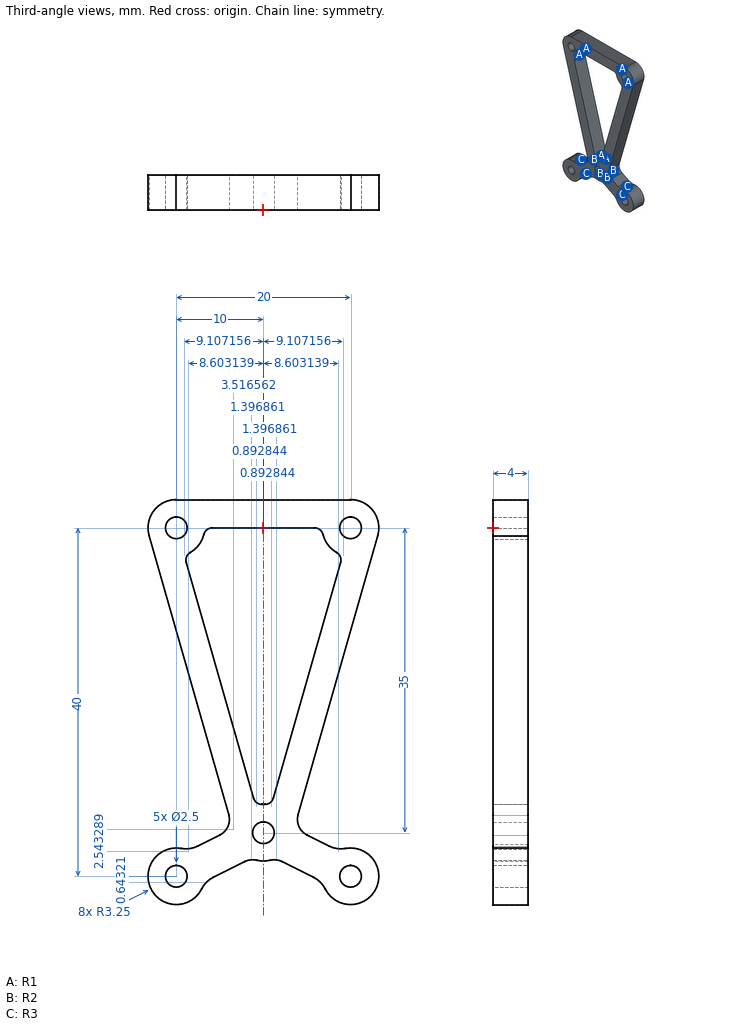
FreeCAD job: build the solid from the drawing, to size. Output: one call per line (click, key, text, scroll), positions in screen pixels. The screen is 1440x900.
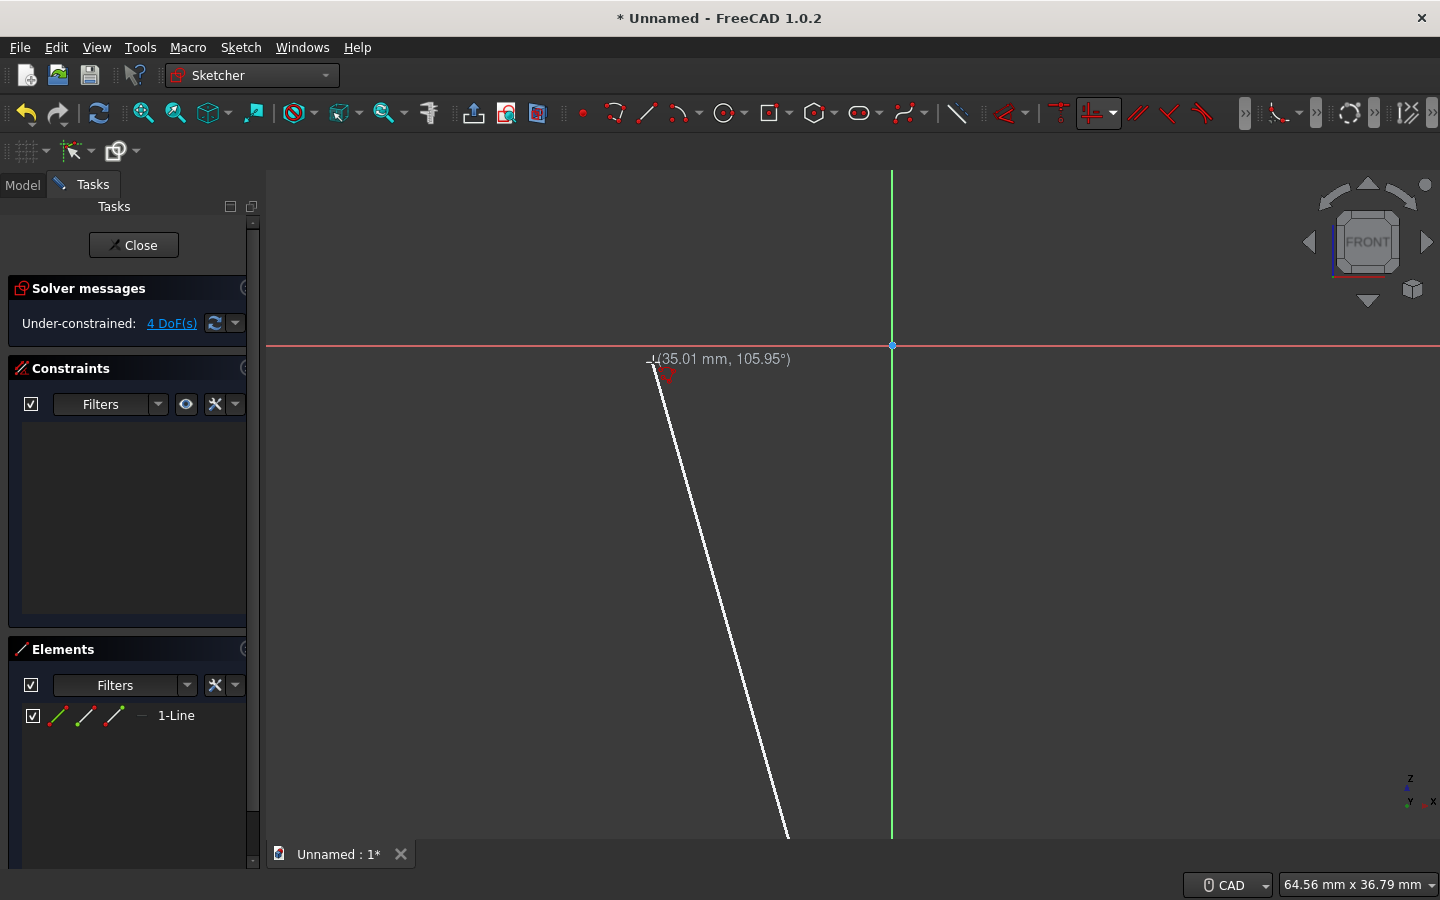
click(653, 362)
right_click(653, 362)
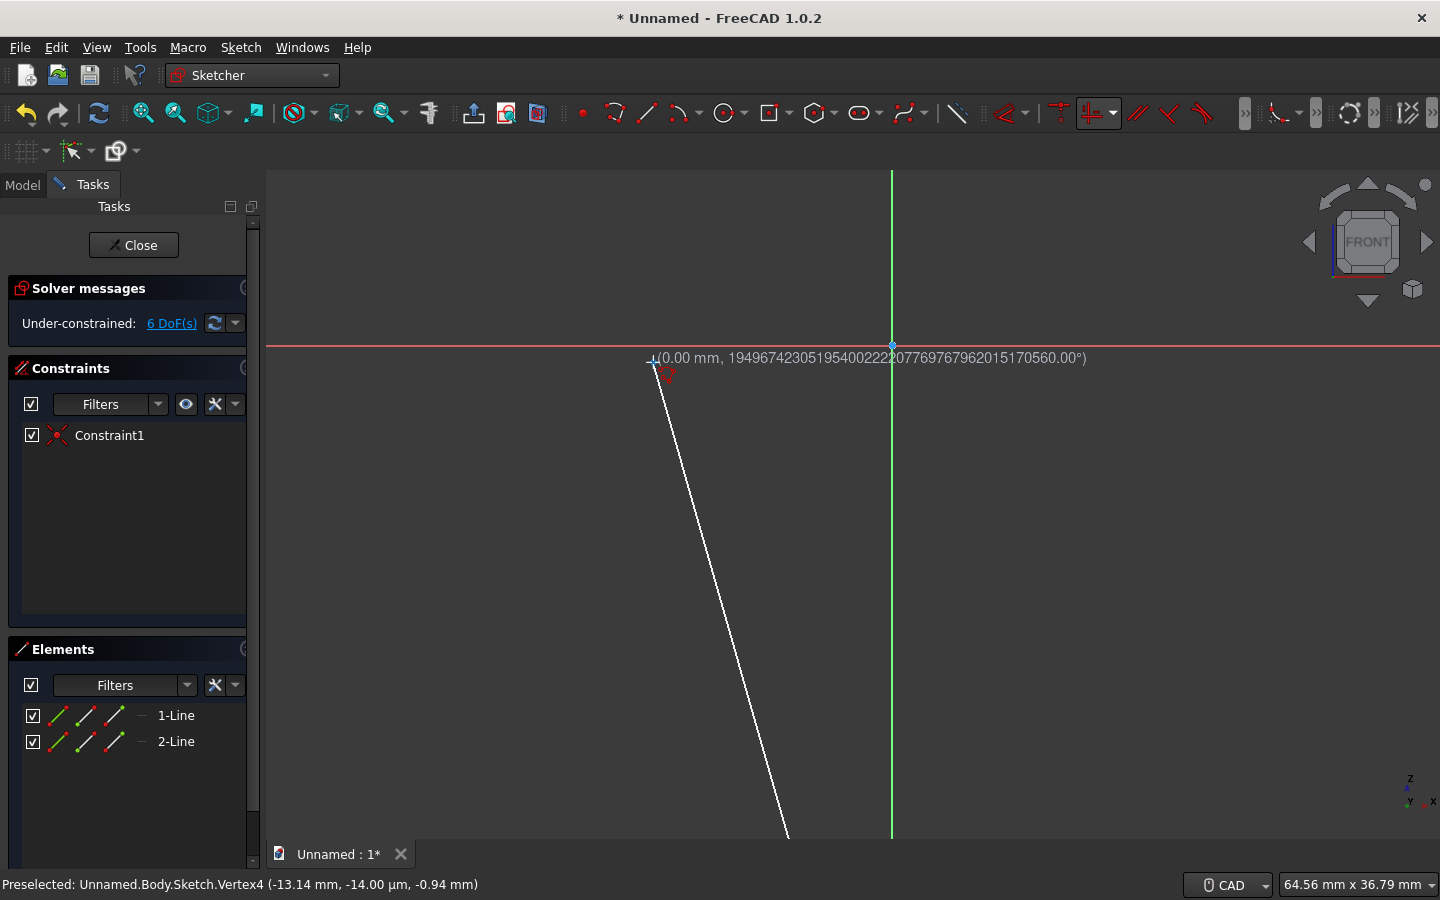
click(648, 114)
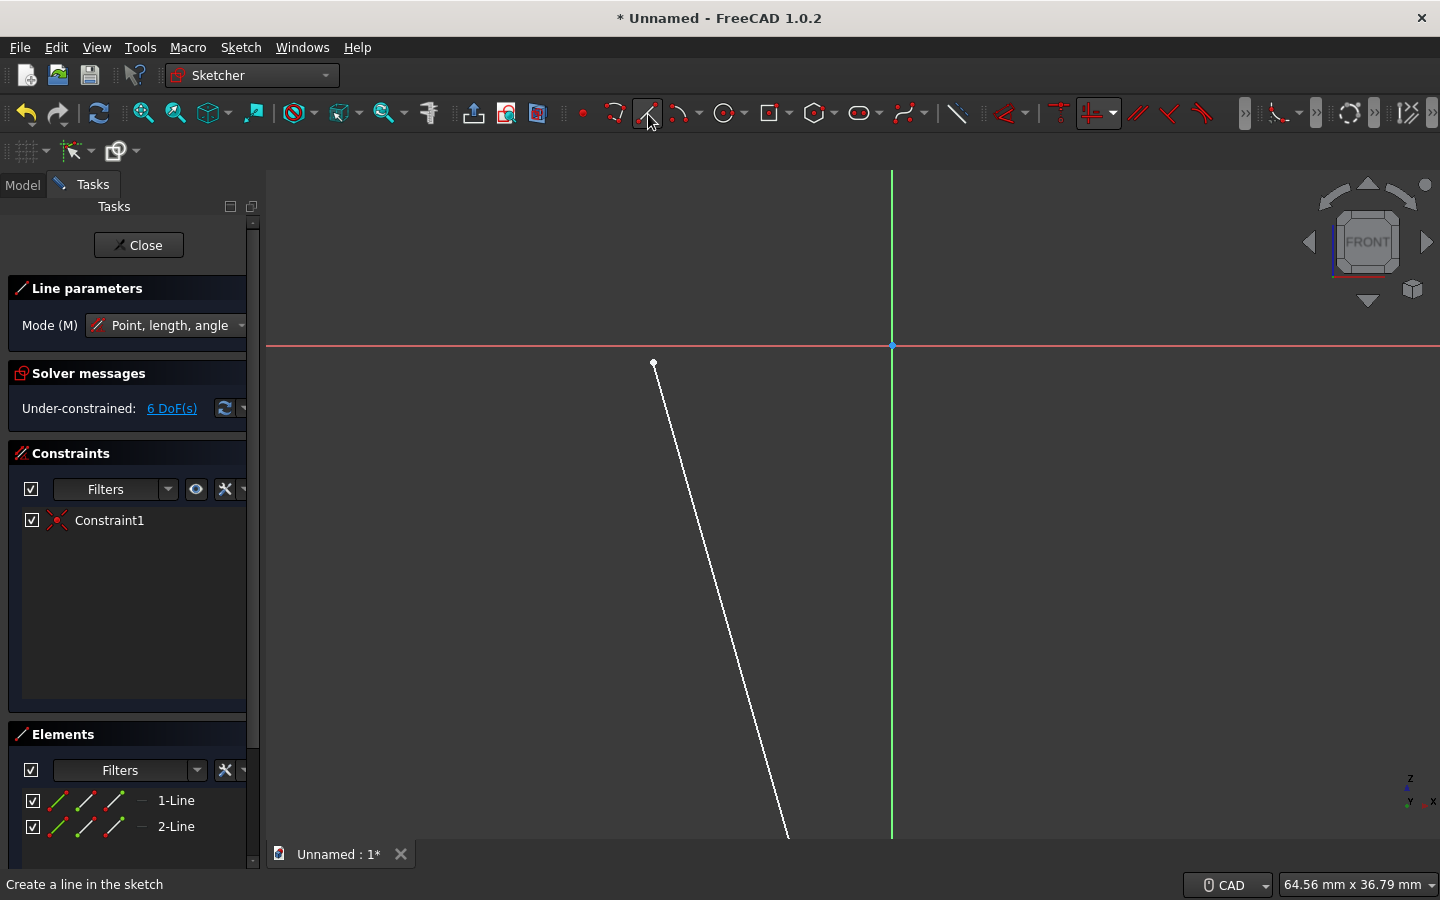
click(710, 287)
click(1074, 287)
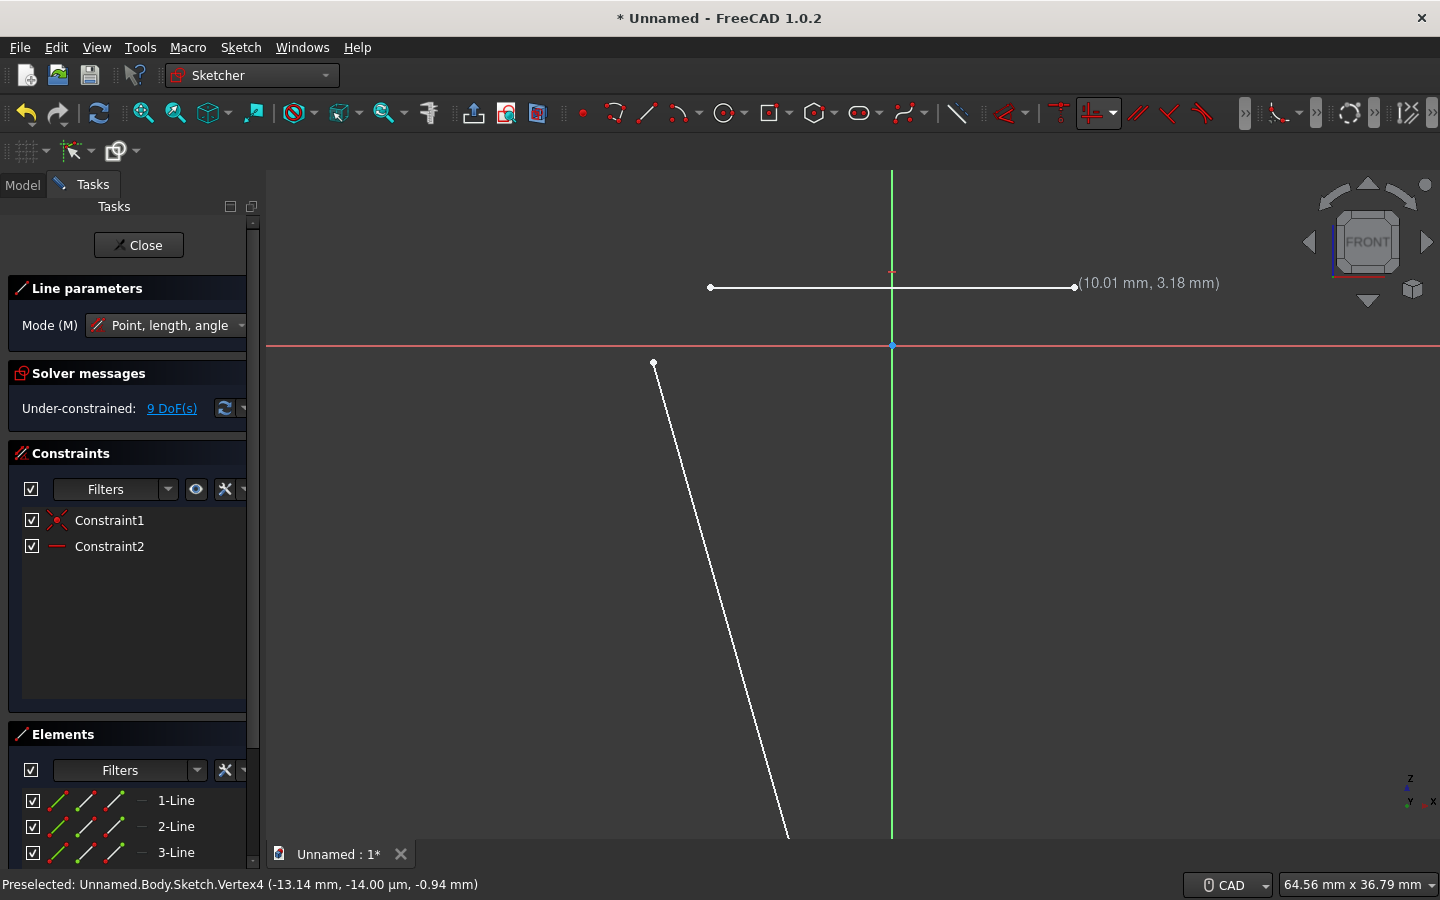
key(g)
key(m)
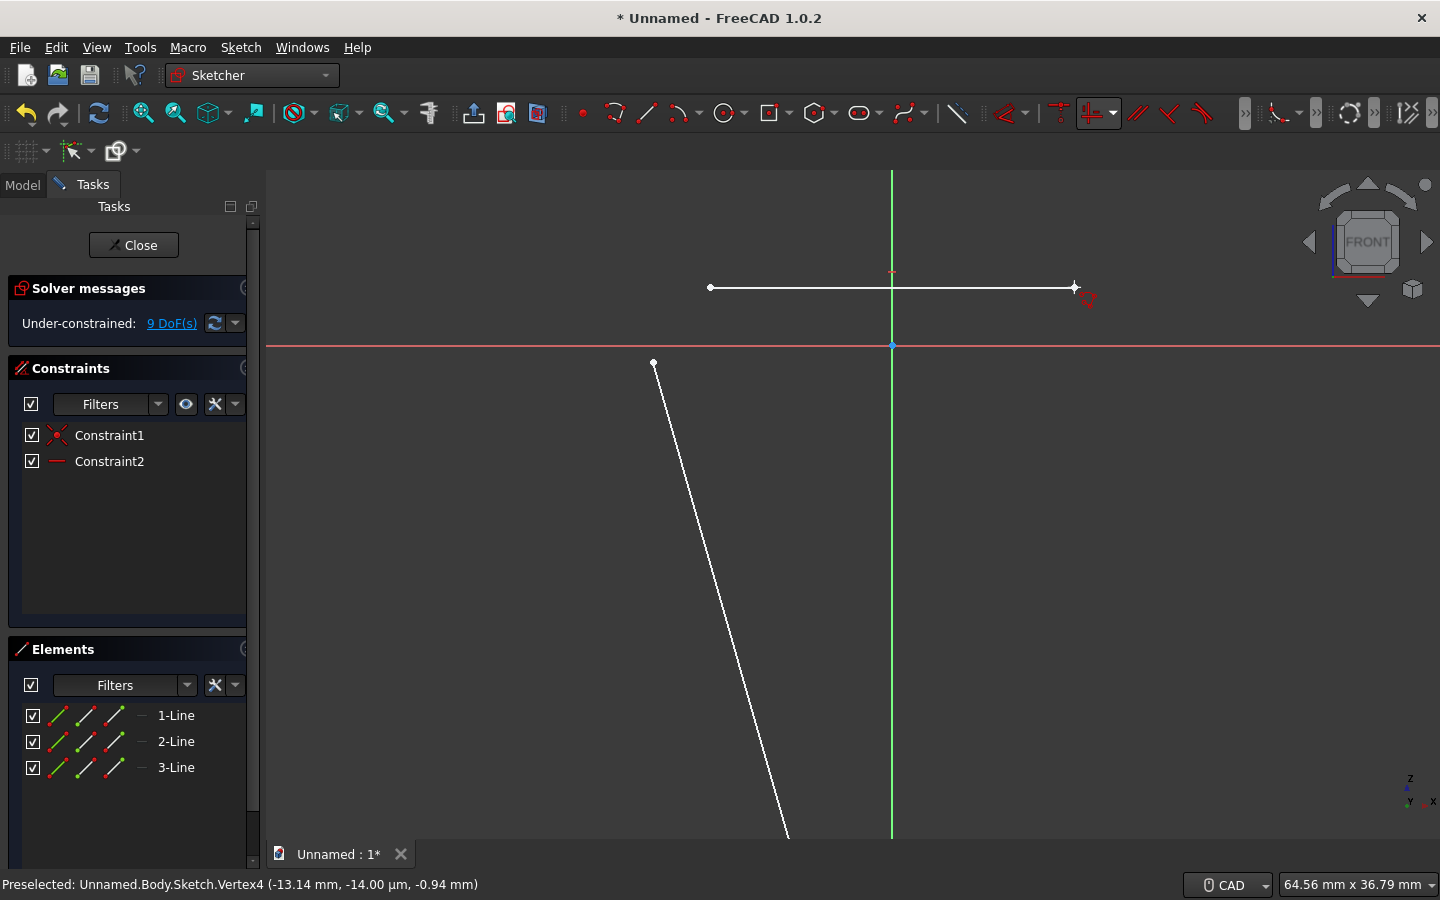
click(1131, 362)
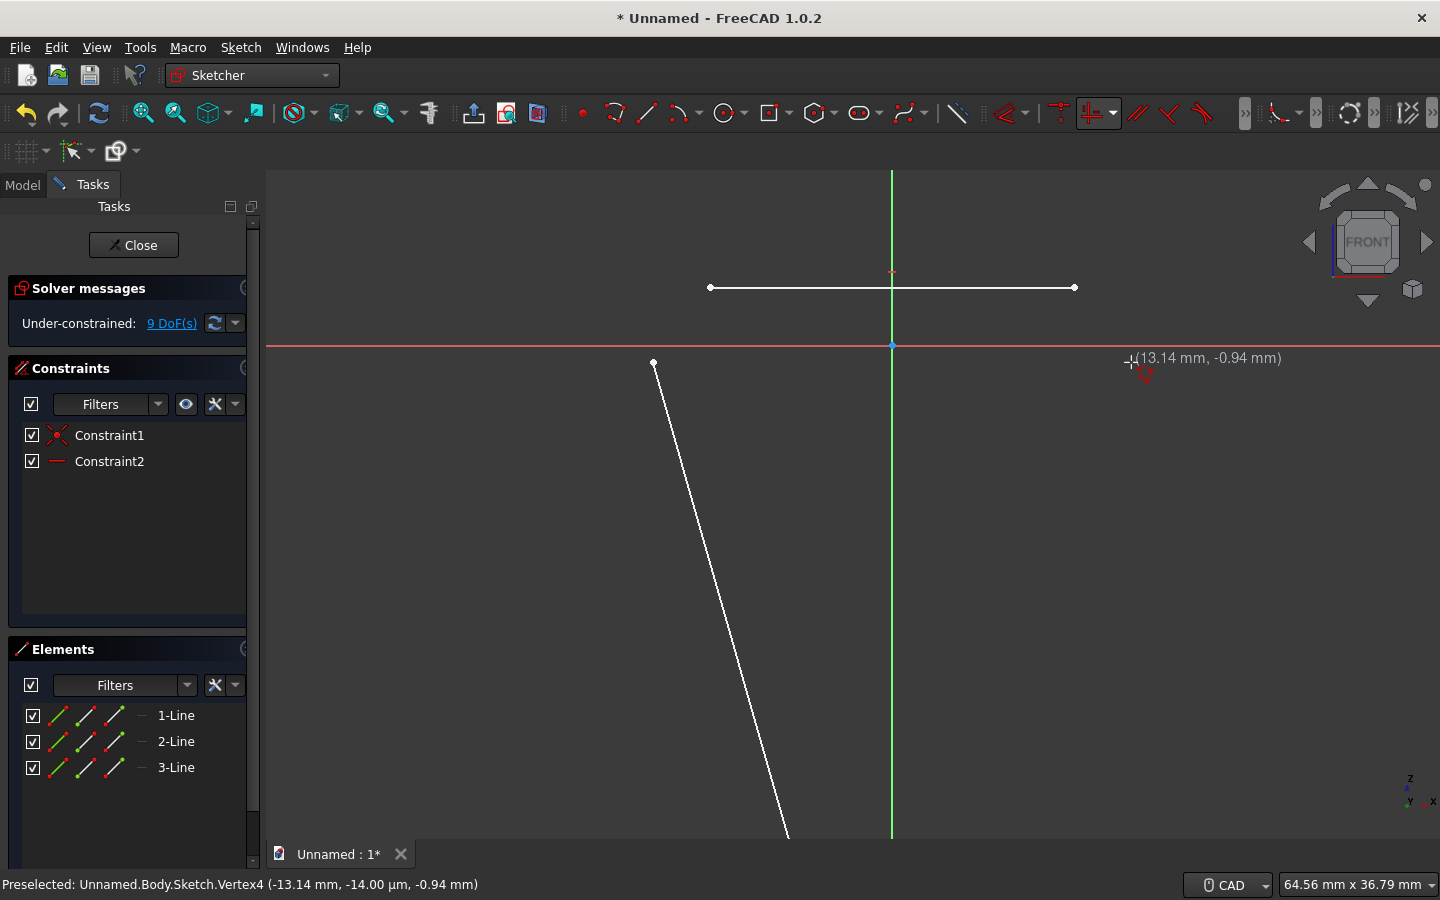
scroll(654, 275, down, 3)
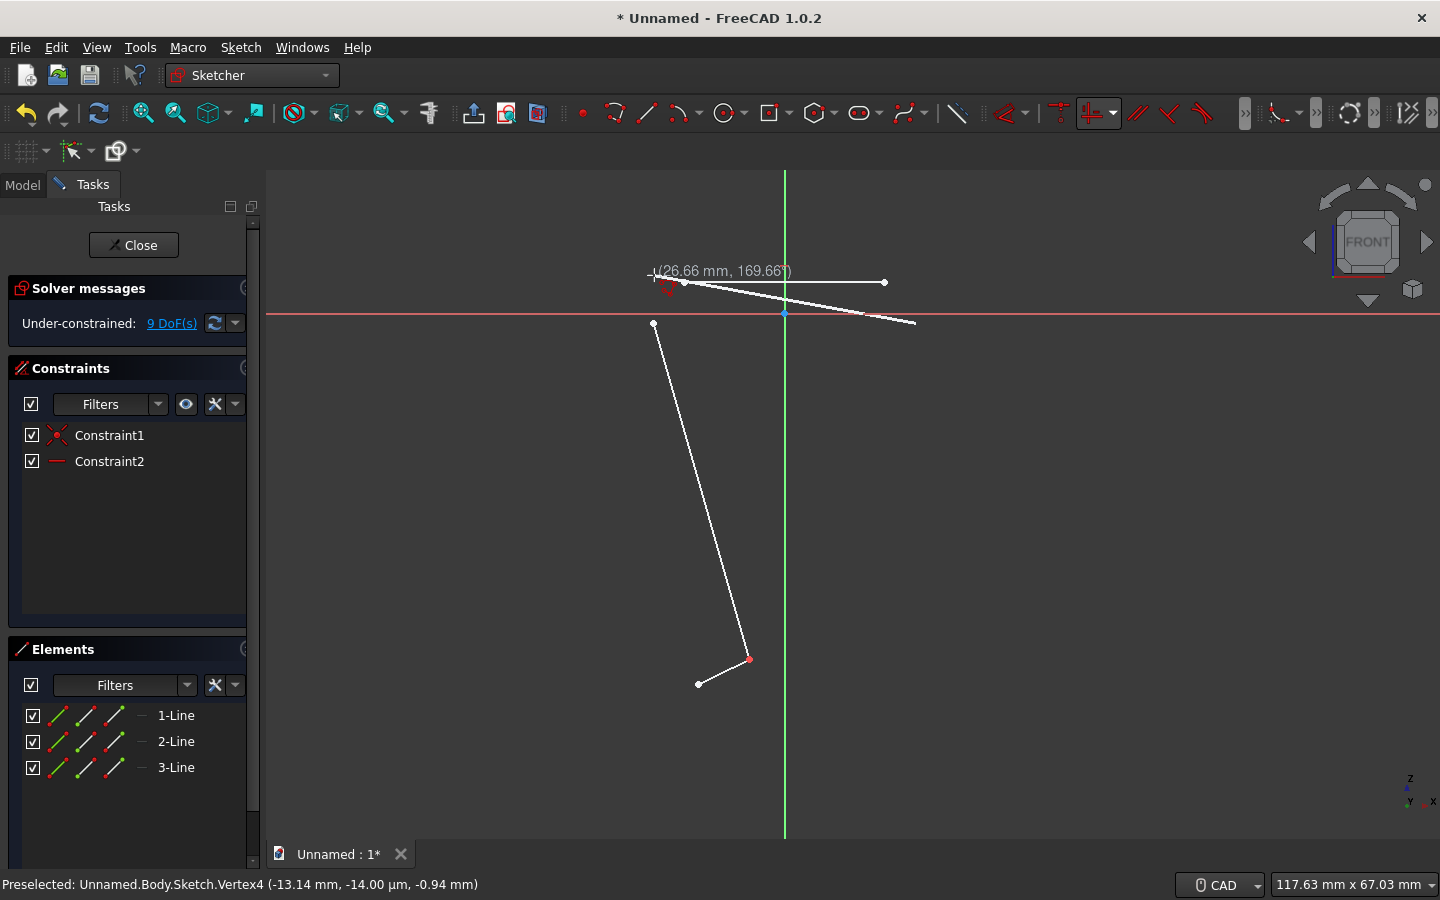
click(820, 659)
click(871, 684)
right_click(871, 684)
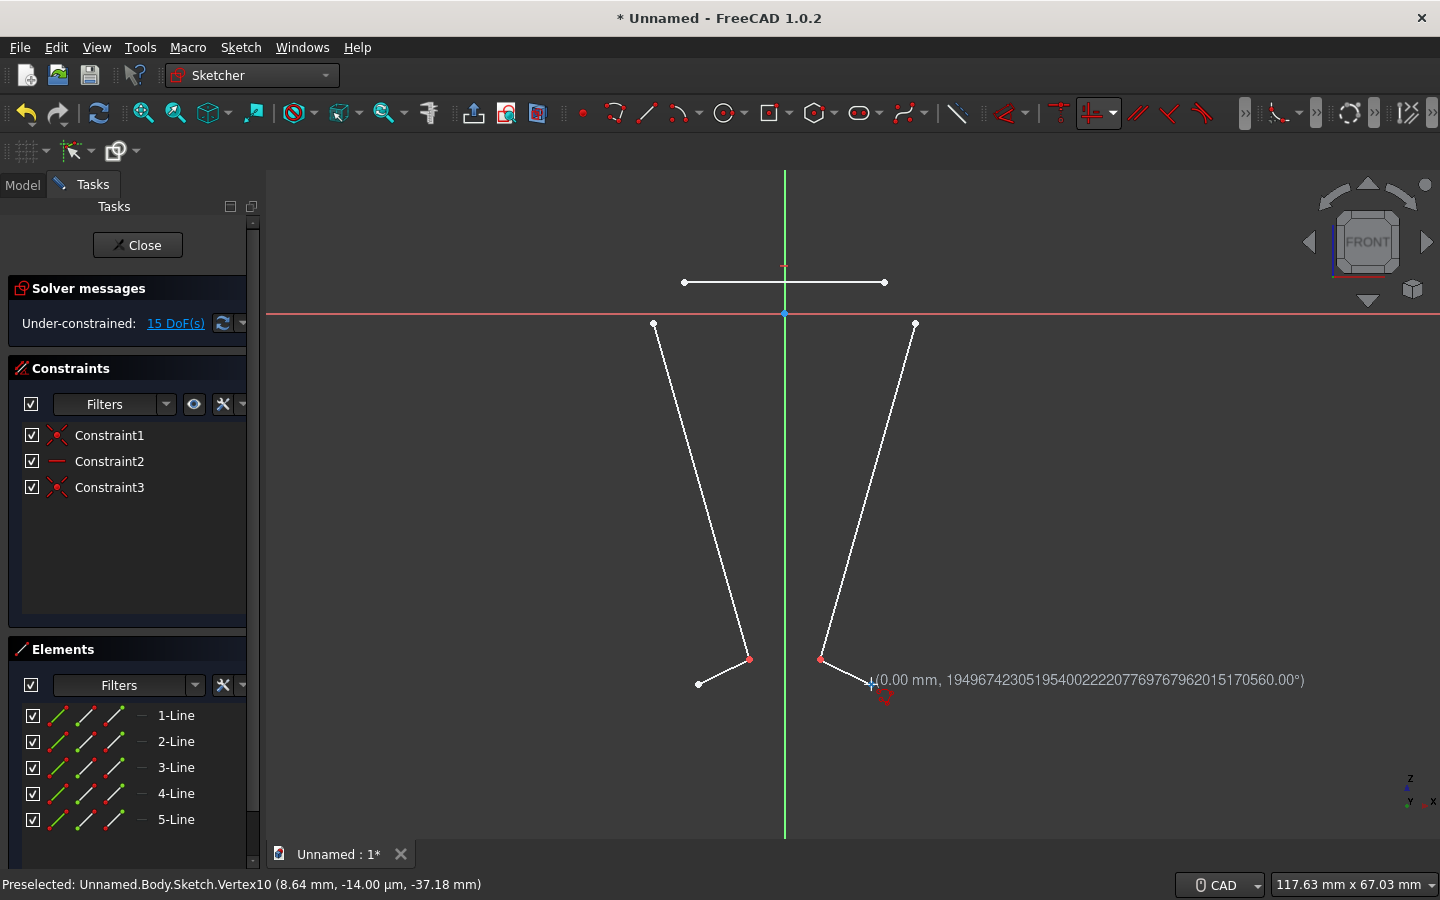
click(648, 114)